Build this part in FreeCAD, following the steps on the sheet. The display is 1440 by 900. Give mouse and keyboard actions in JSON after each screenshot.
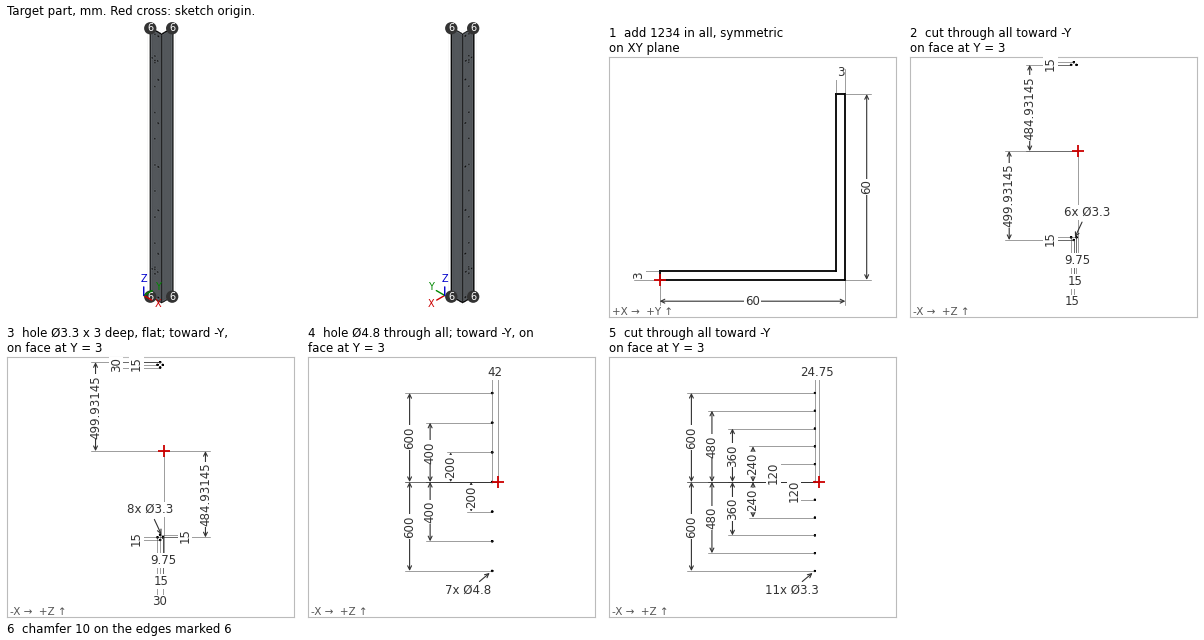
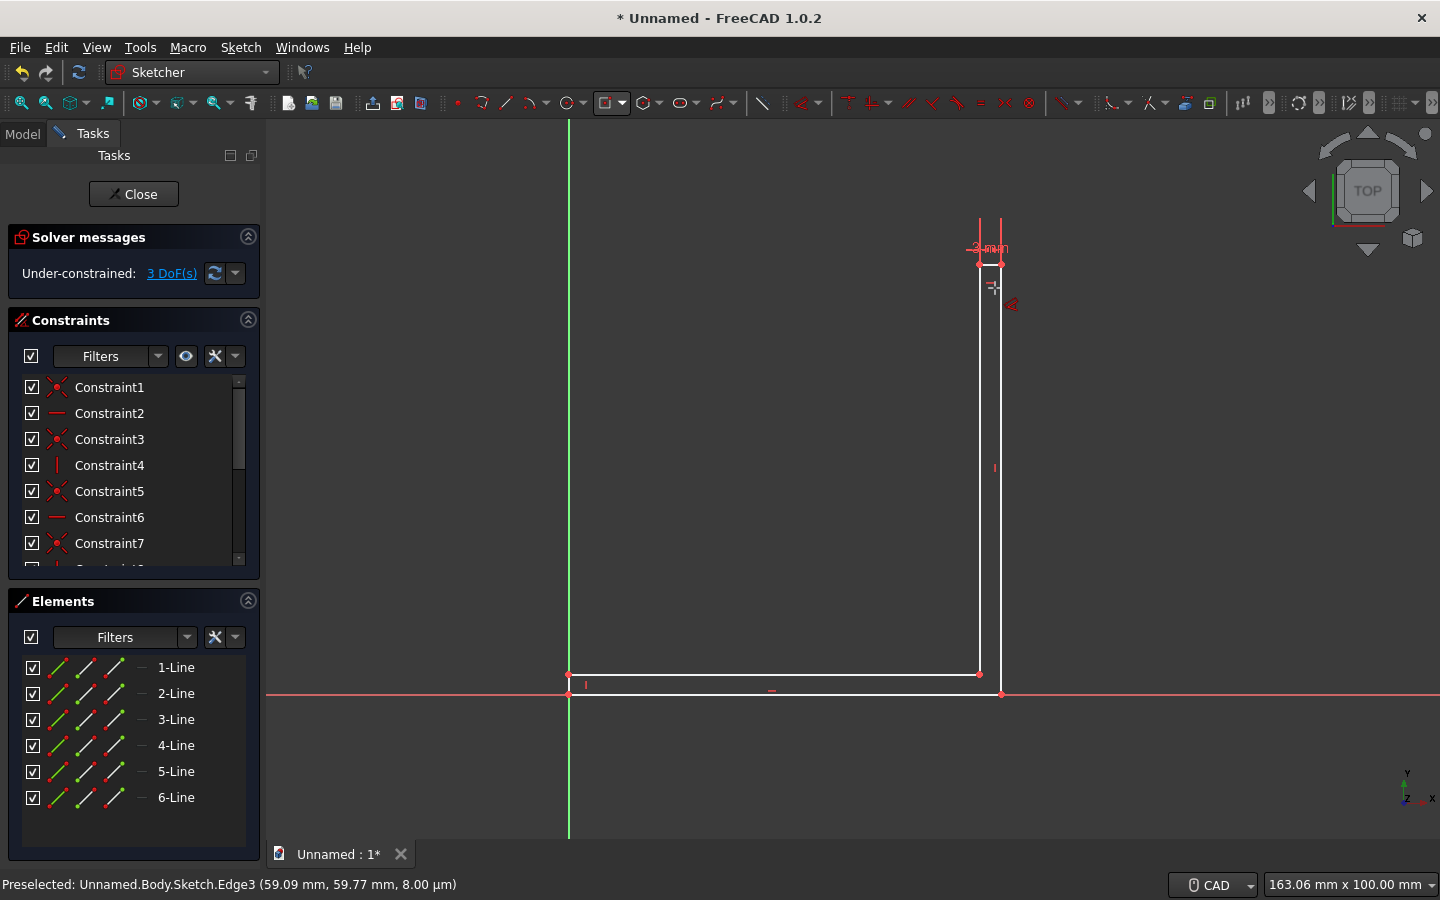
{"action": "scroll", "coordinate": [569, 681], "scroll_direction": "up", "scroll_amount": 5}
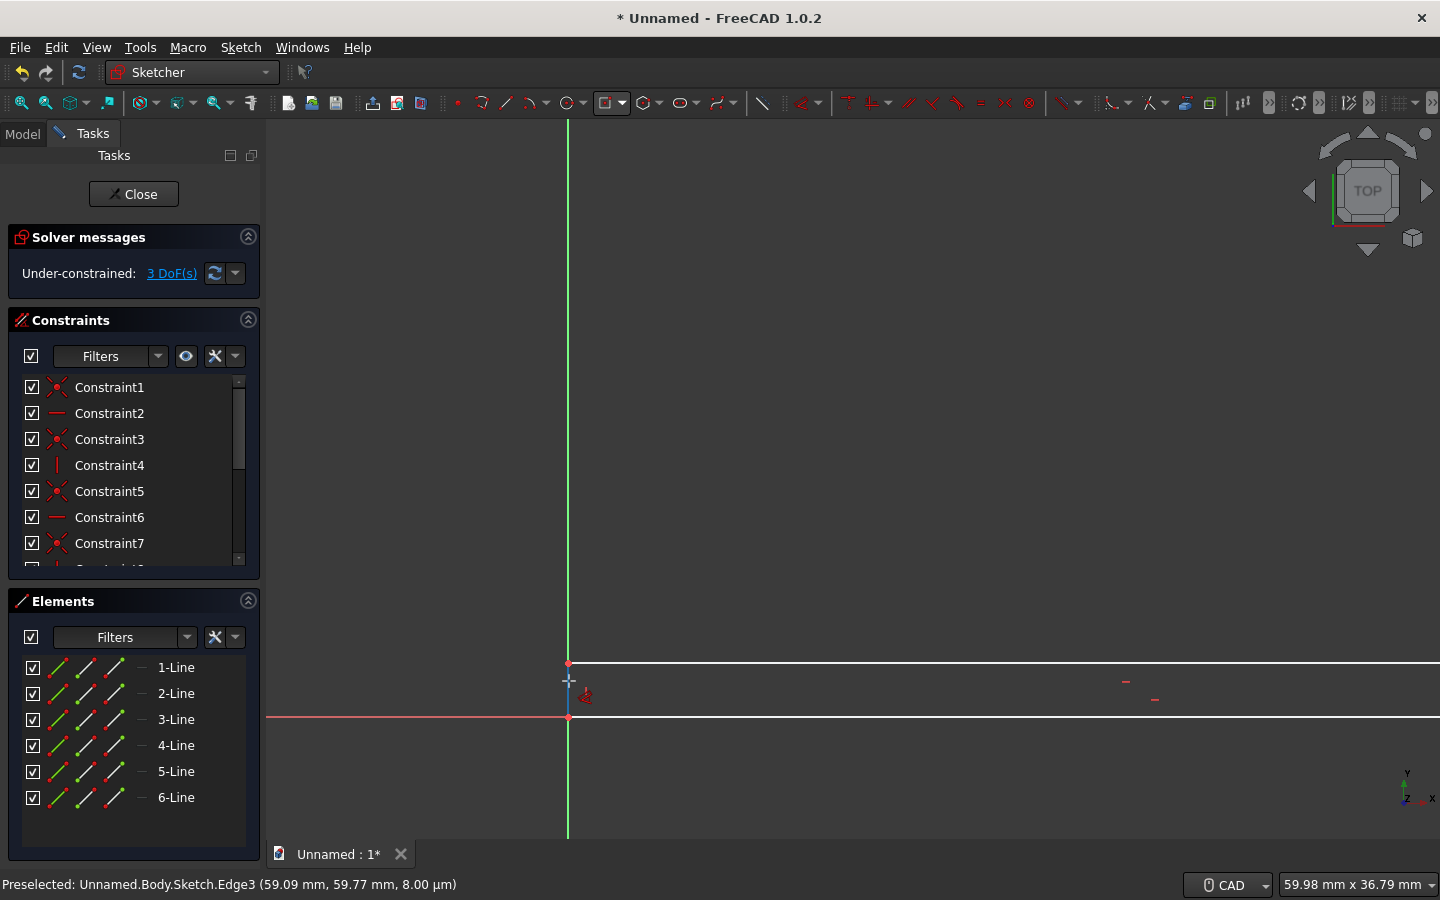
{"action": "left_click", "coordinate": [568, 679]}
{"action": "left_click", "coordinate": [534, 690]}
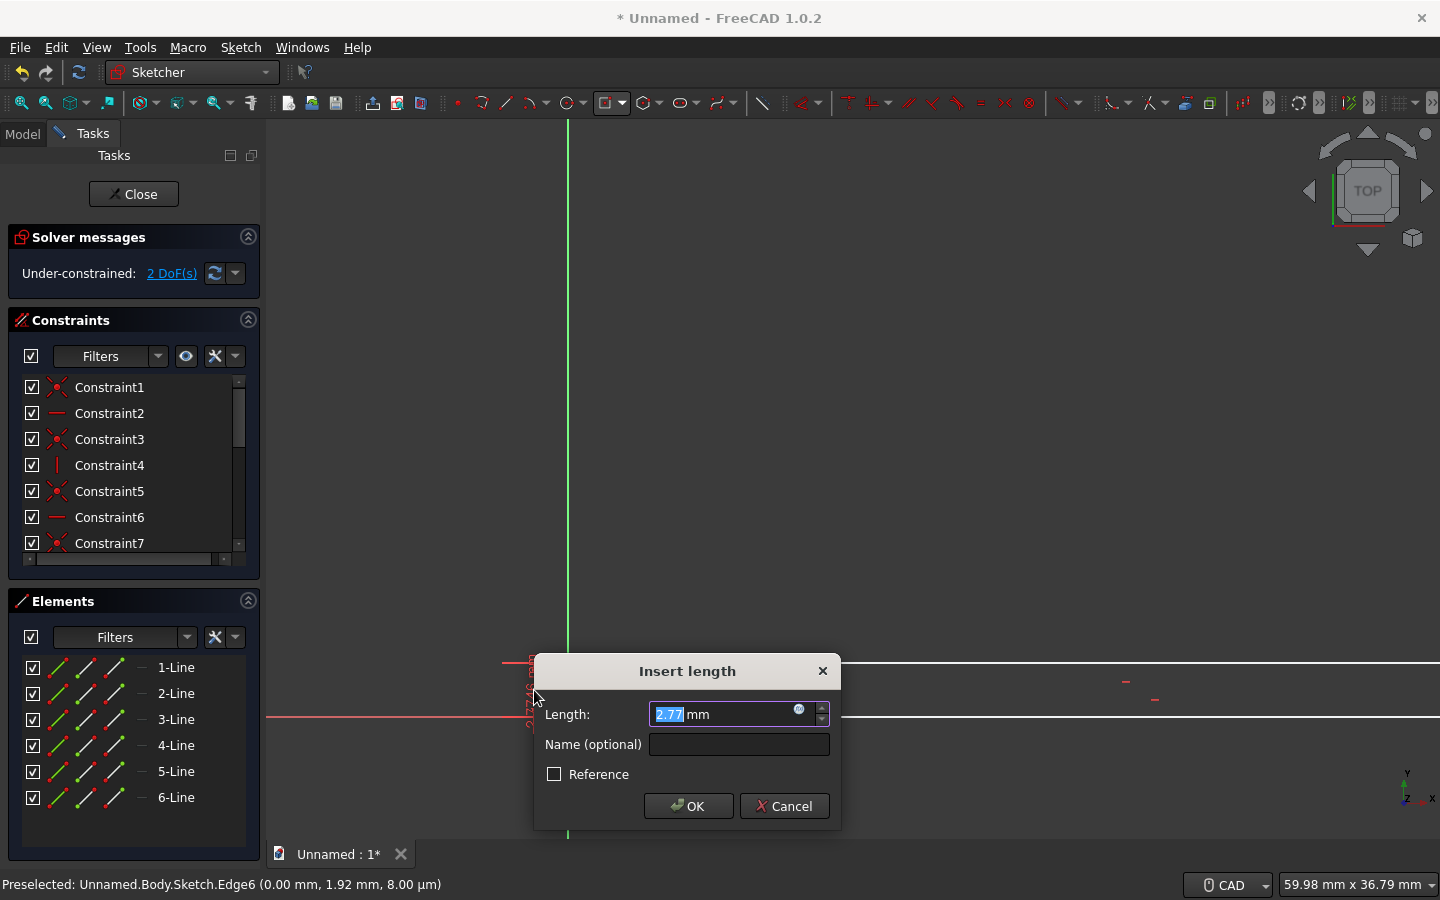
{"action": "type", "text": "3"}
{"action": "key", "text": "Return"}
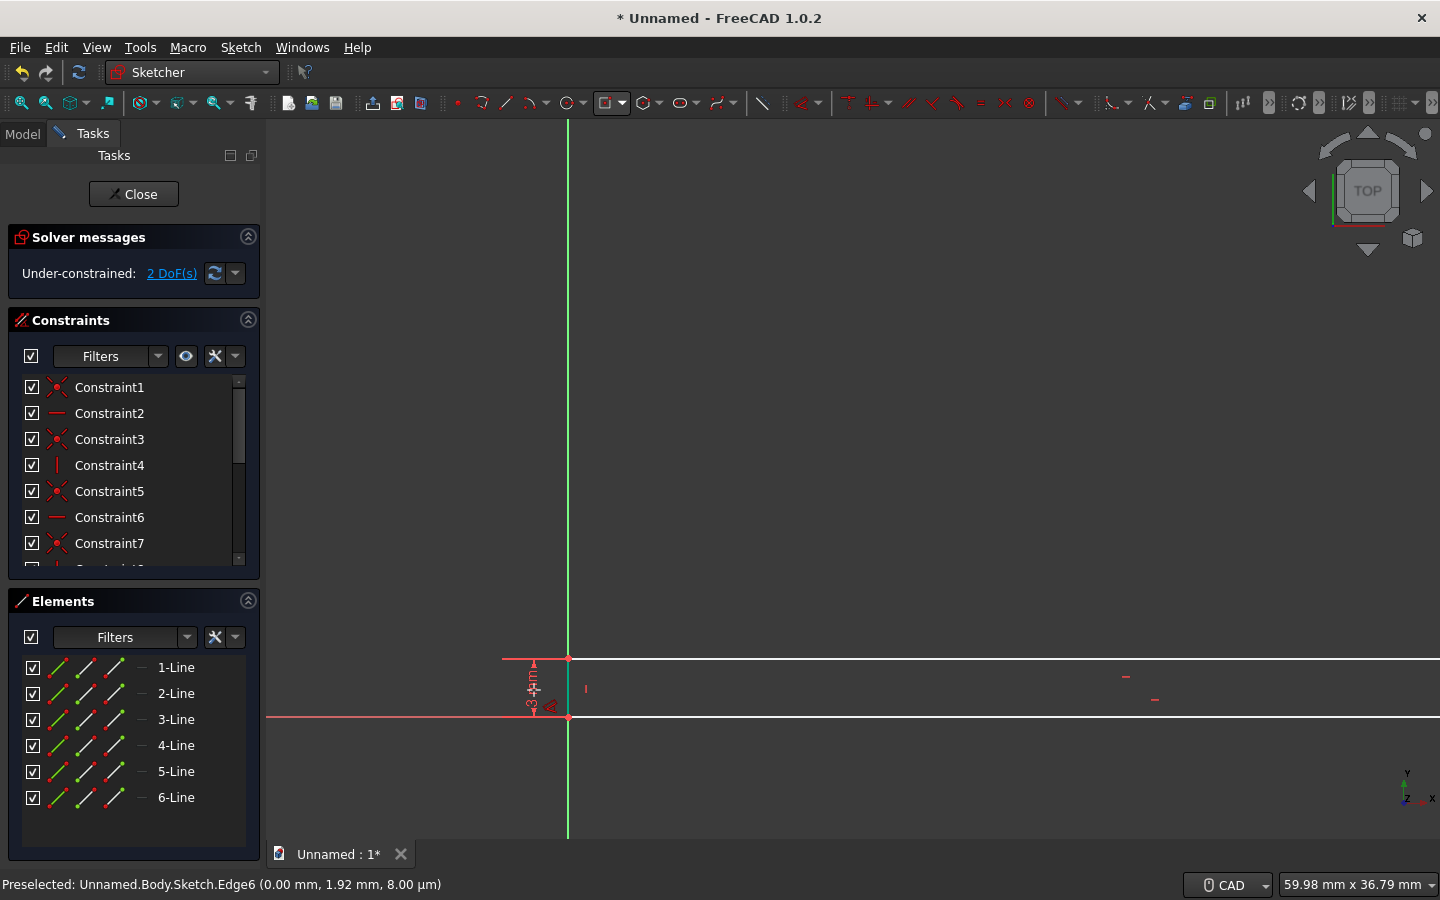
{"action": "left_click", "coordinate": [921, 717]}
{"action": "left_click", "coordinate": [922, 751]}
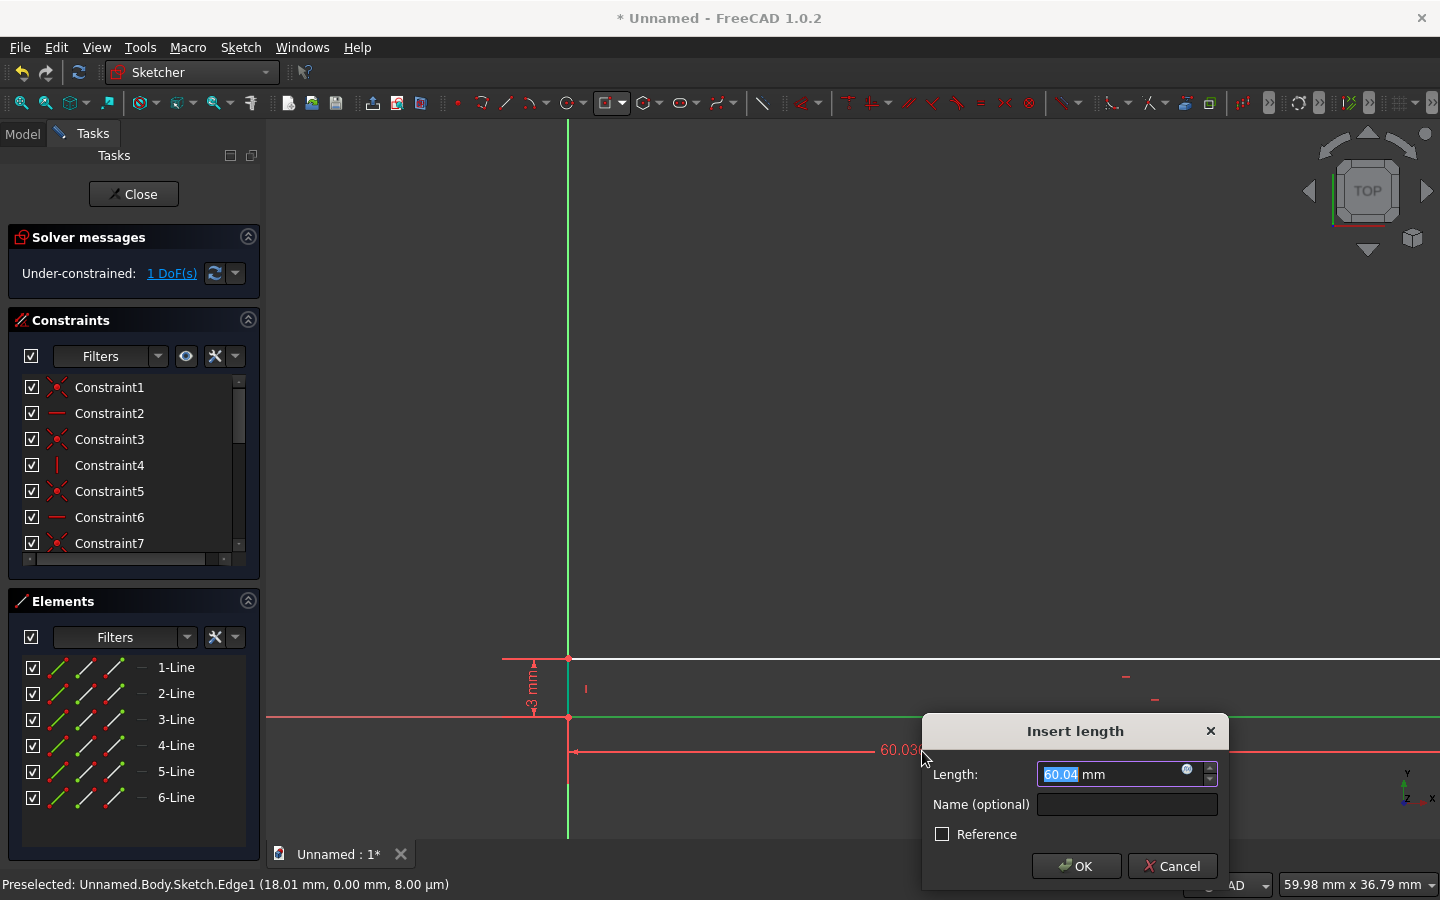
{"action": "type", "text": "60"}
{"action": "key", "text": "Return"}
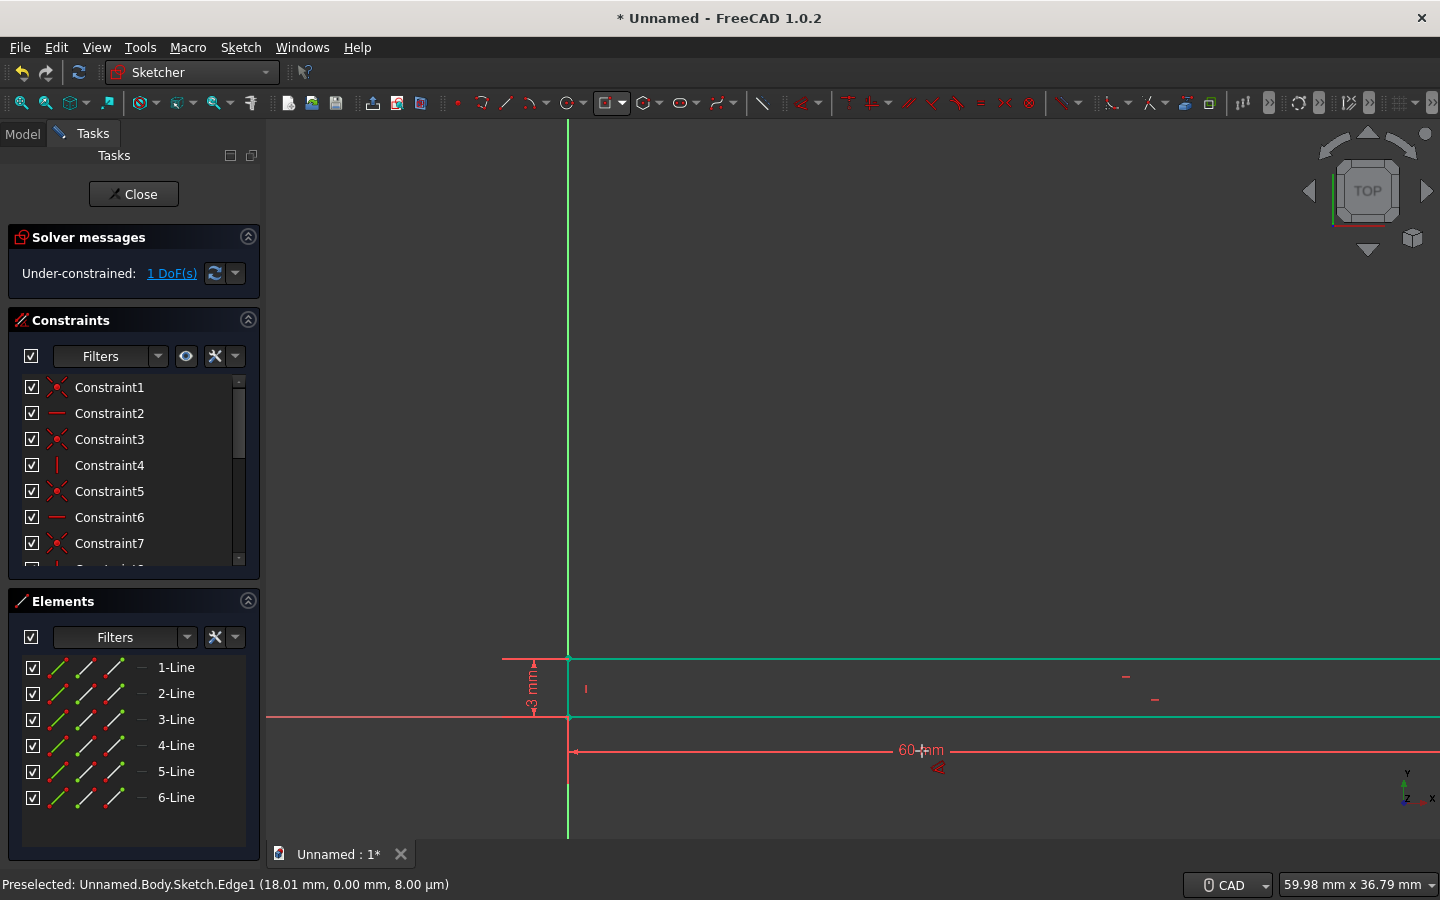
{"action": "scroll", "coordinate": [569, 682], "scroll_direction": "down", "scroll_amount": 5}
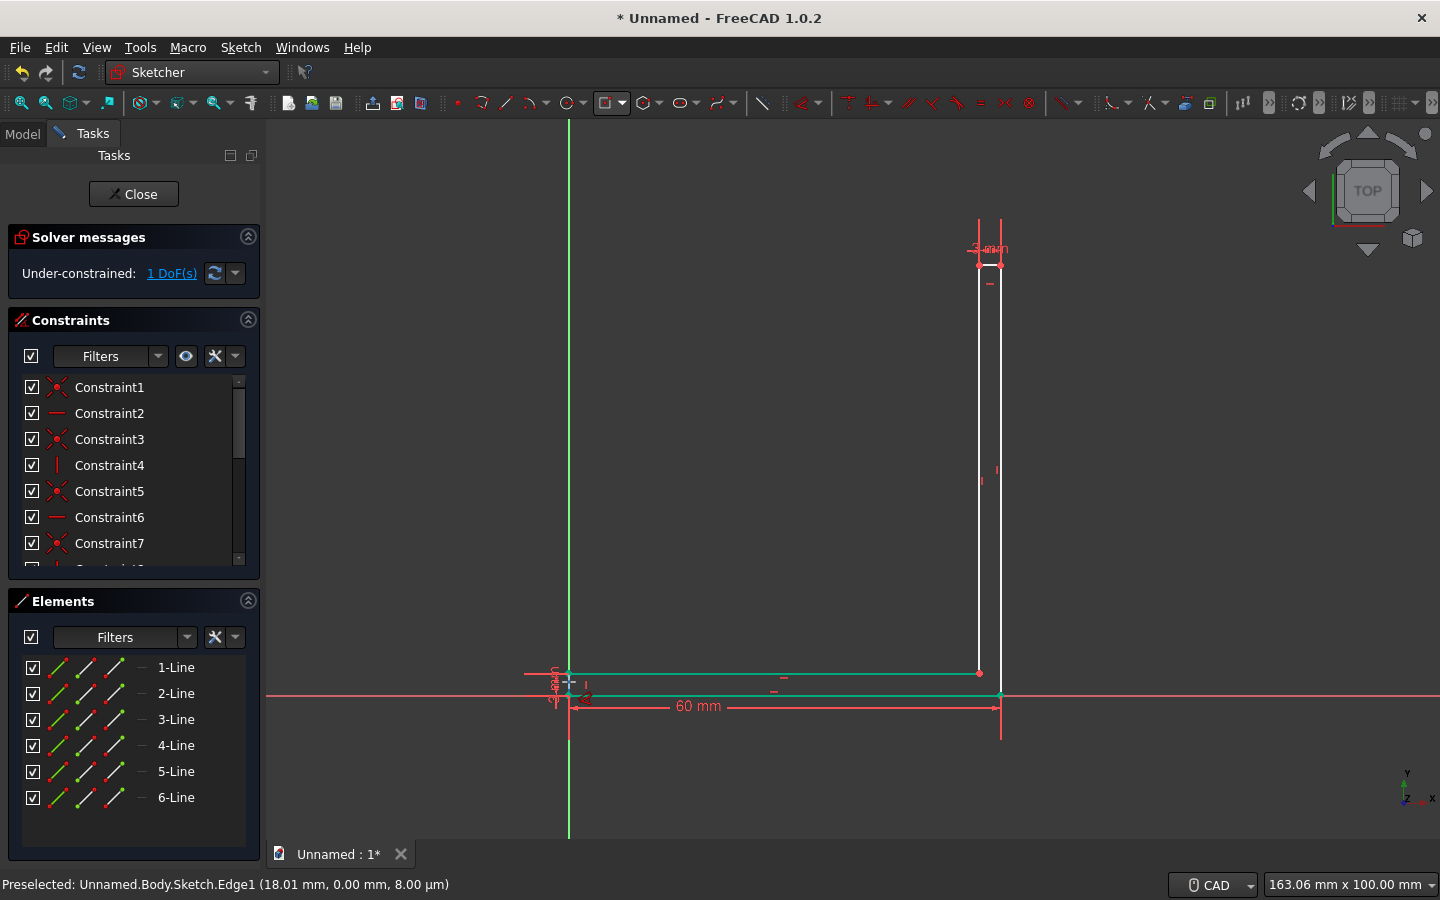
{"action": "left_click", "coordinate": [1001, 566]}
{"action": "left_click", "coordinate": [1035, 480]}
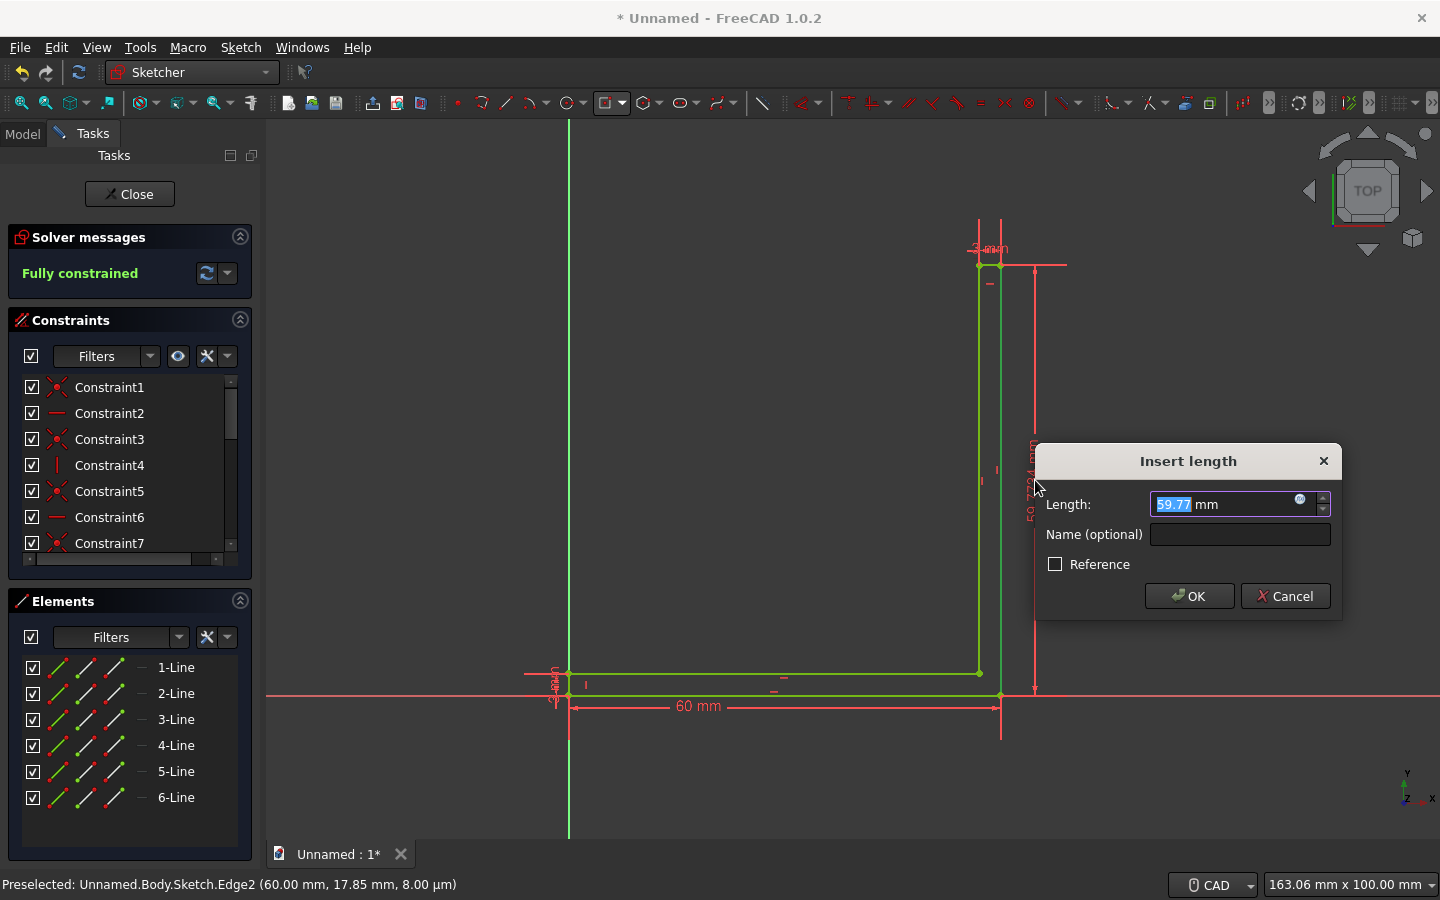
{"action": "type", "text": "60"}
{"action": "key", "text": "Return"}
{"action": "key", "text": "Escape"}